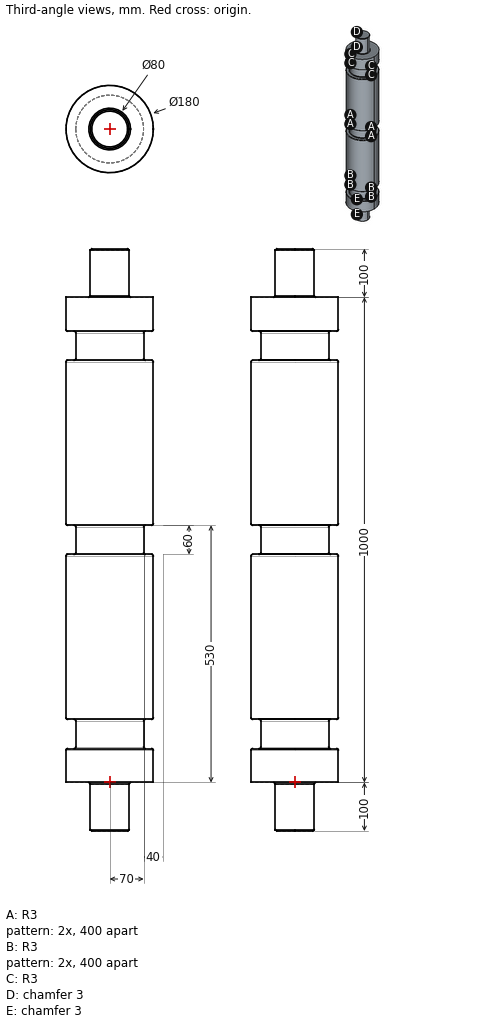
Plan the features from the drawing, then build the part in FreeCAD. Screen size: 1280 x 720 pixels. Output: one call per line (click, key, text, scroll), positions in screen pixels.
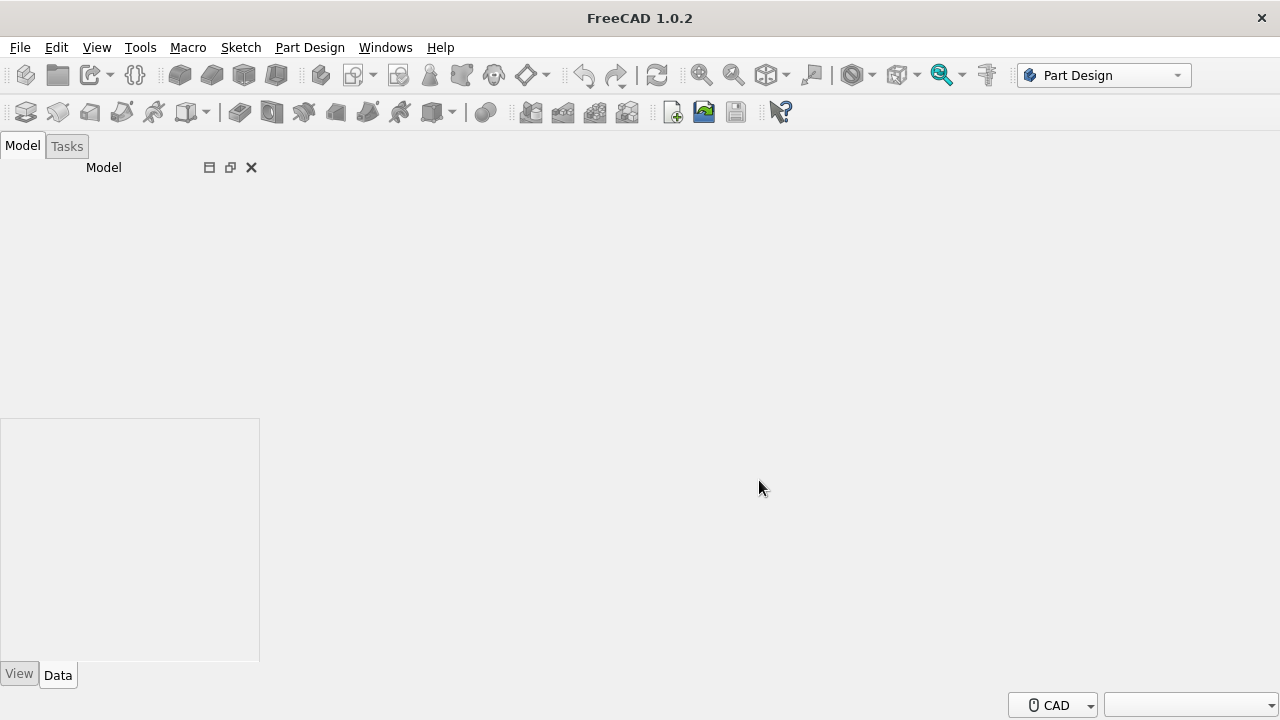
click(672, 112)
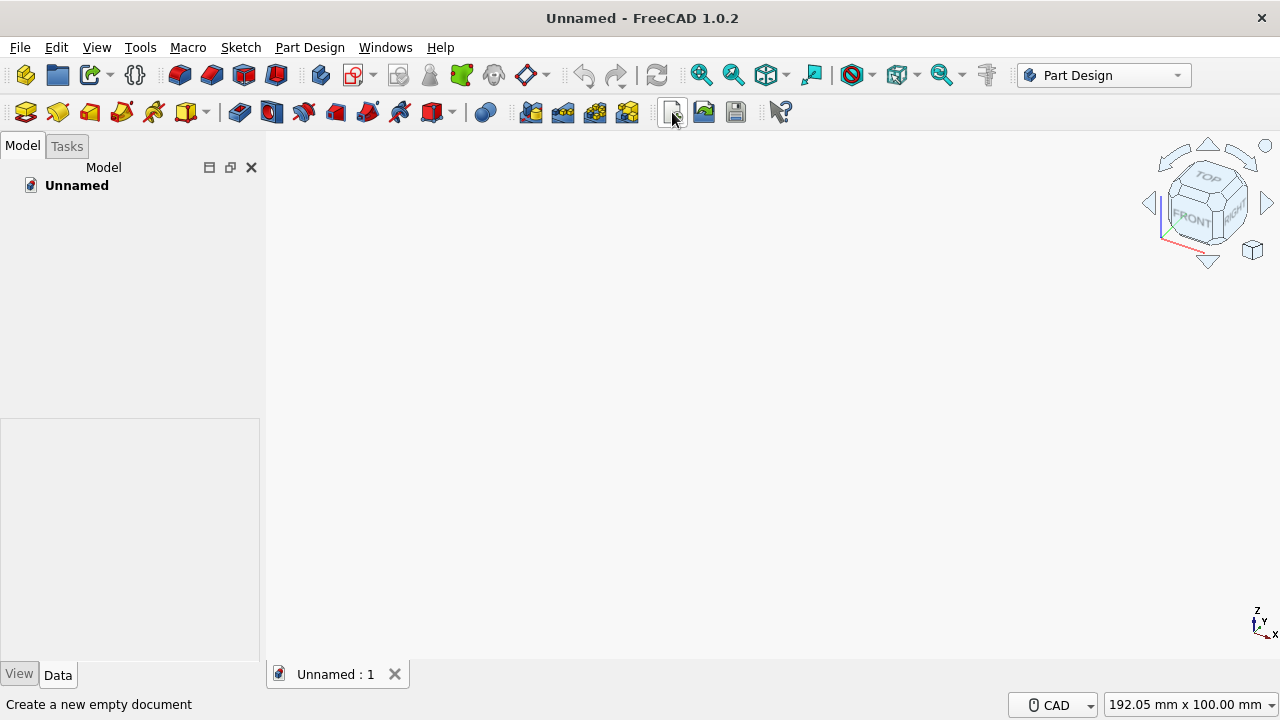
click(354, 76)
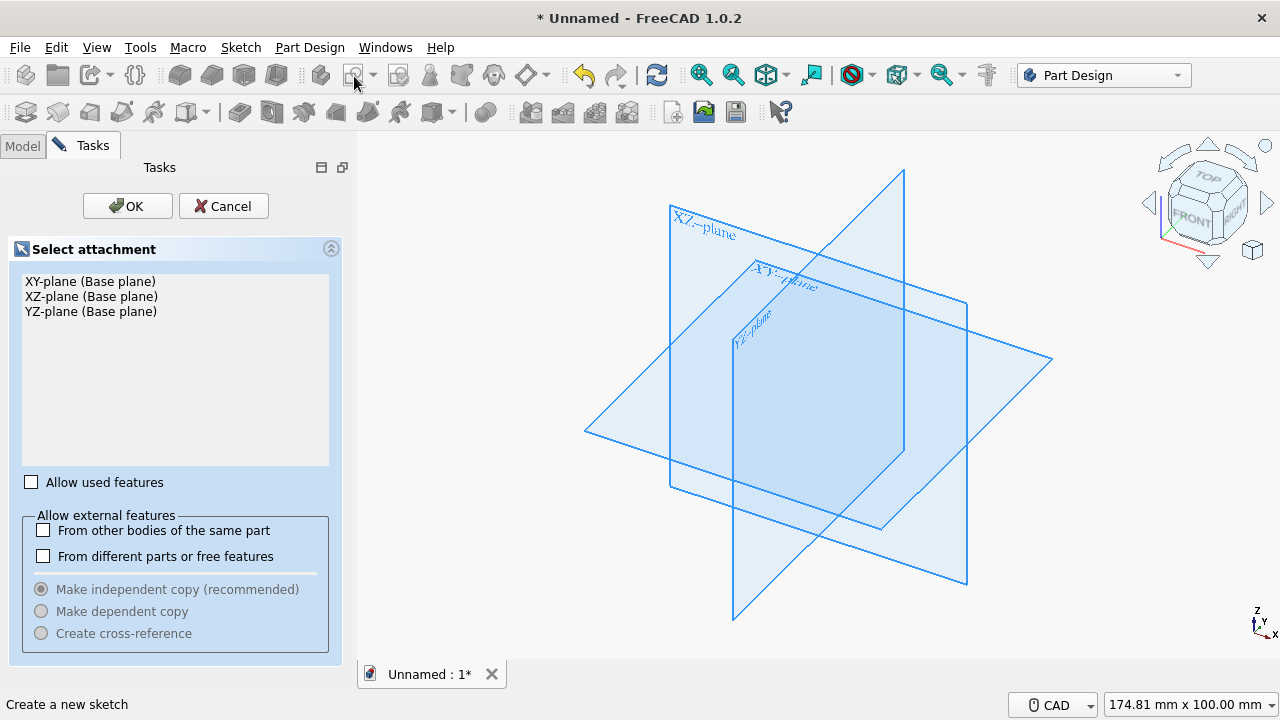
click(82, 282)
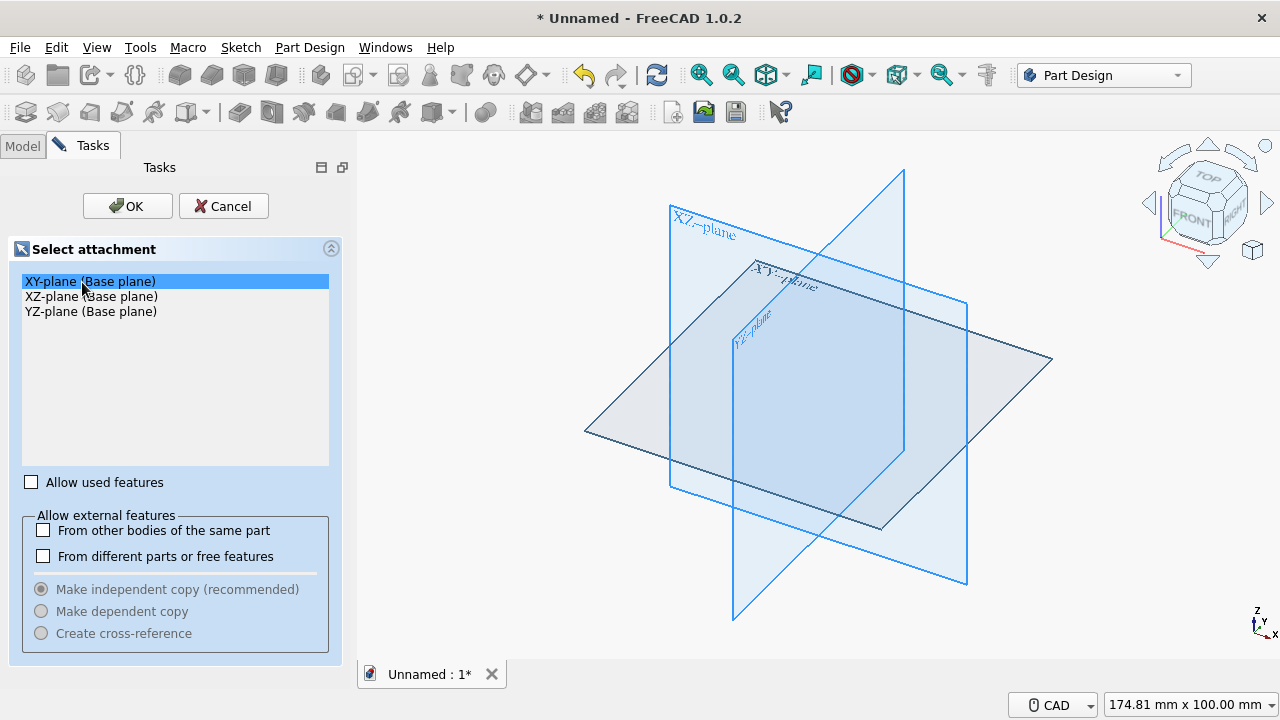
click(128, 206)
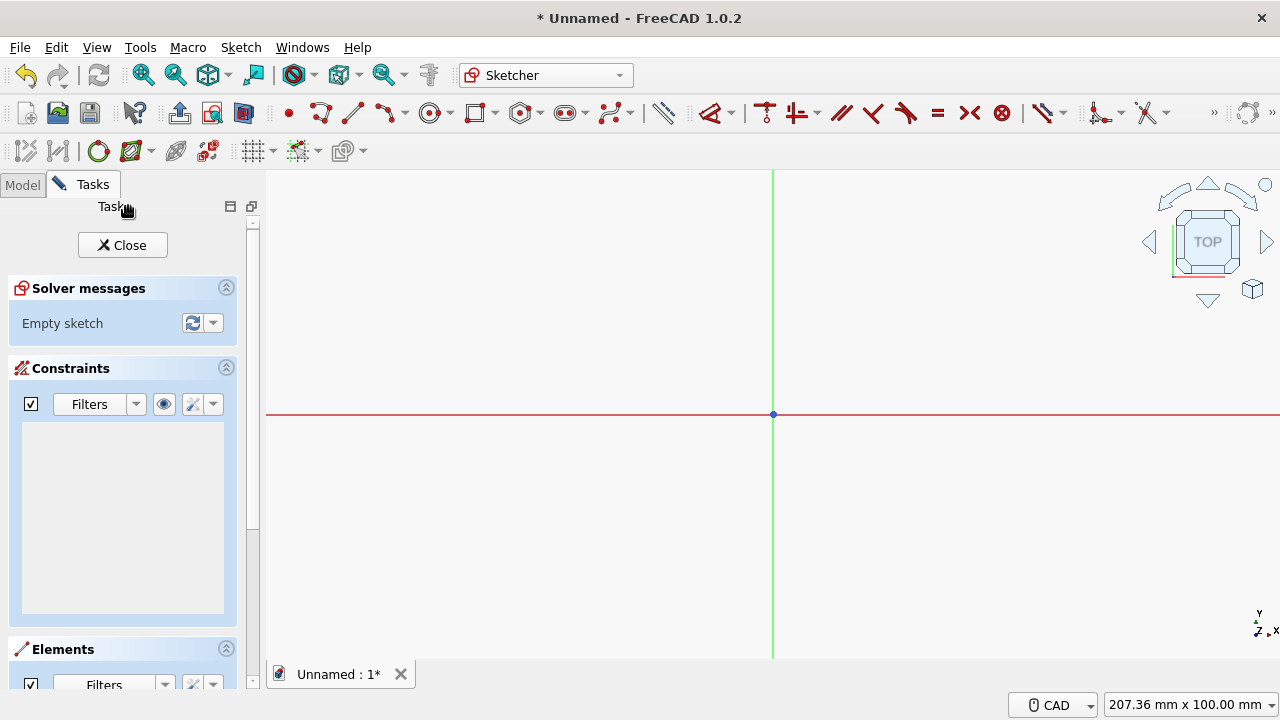
scroll(665, 414, down, 5)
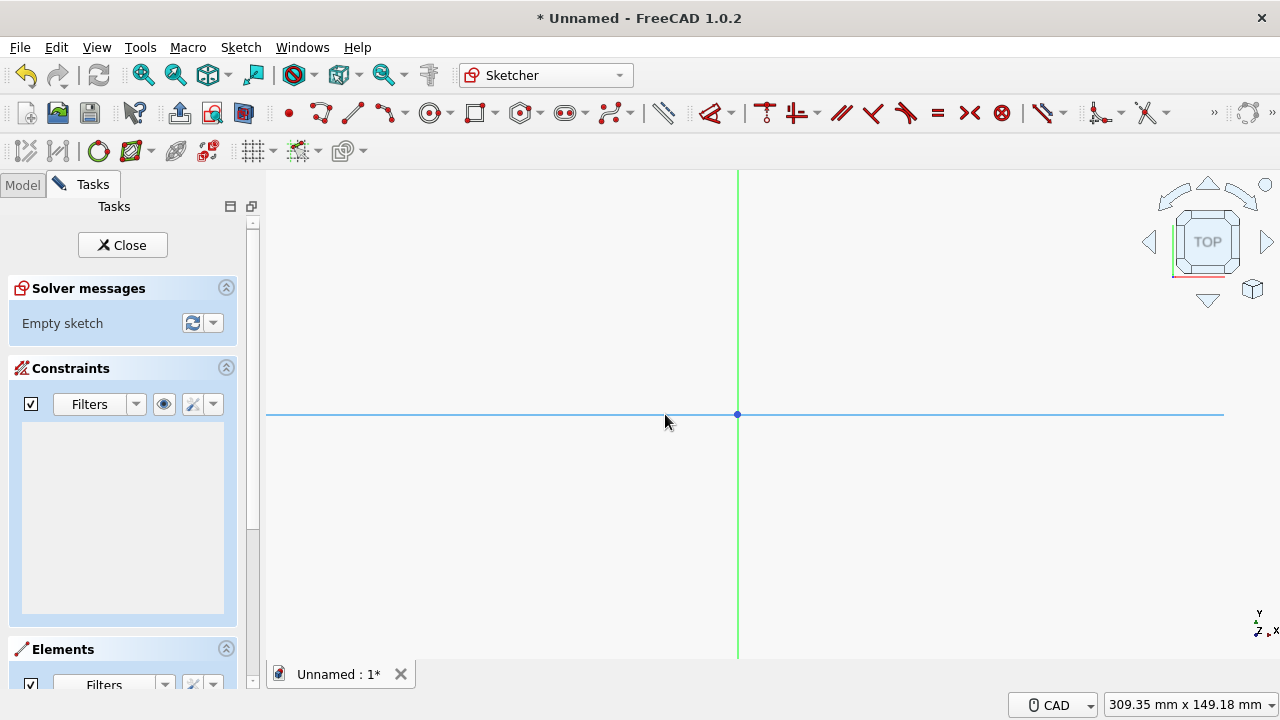
click(430, 114)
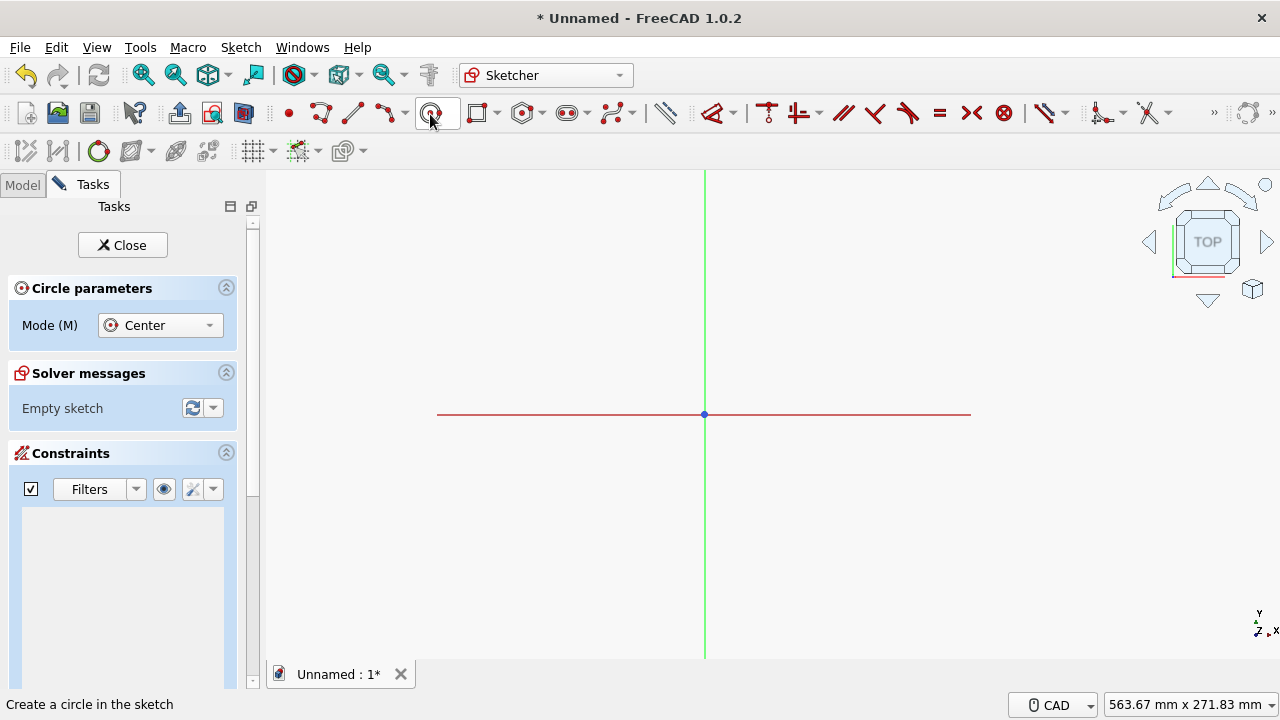
click(705, 414)
move(819, 300)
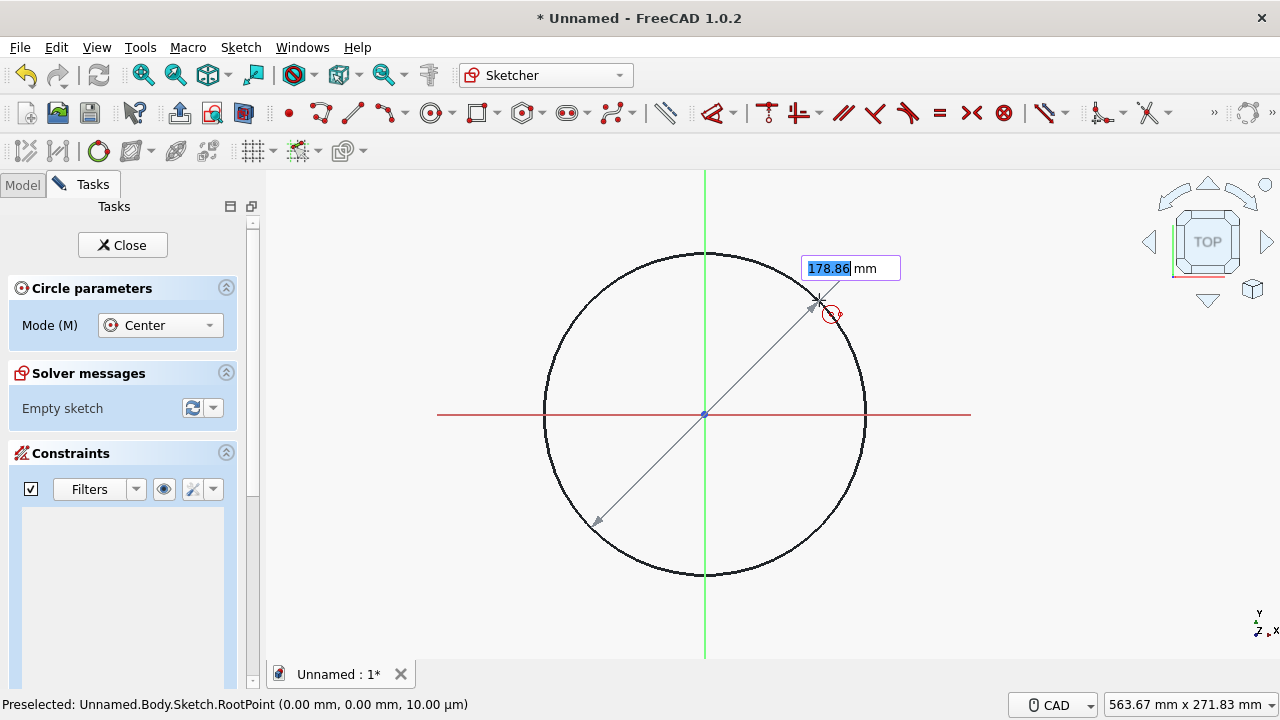
text(180)
key(Return)
key(Escape)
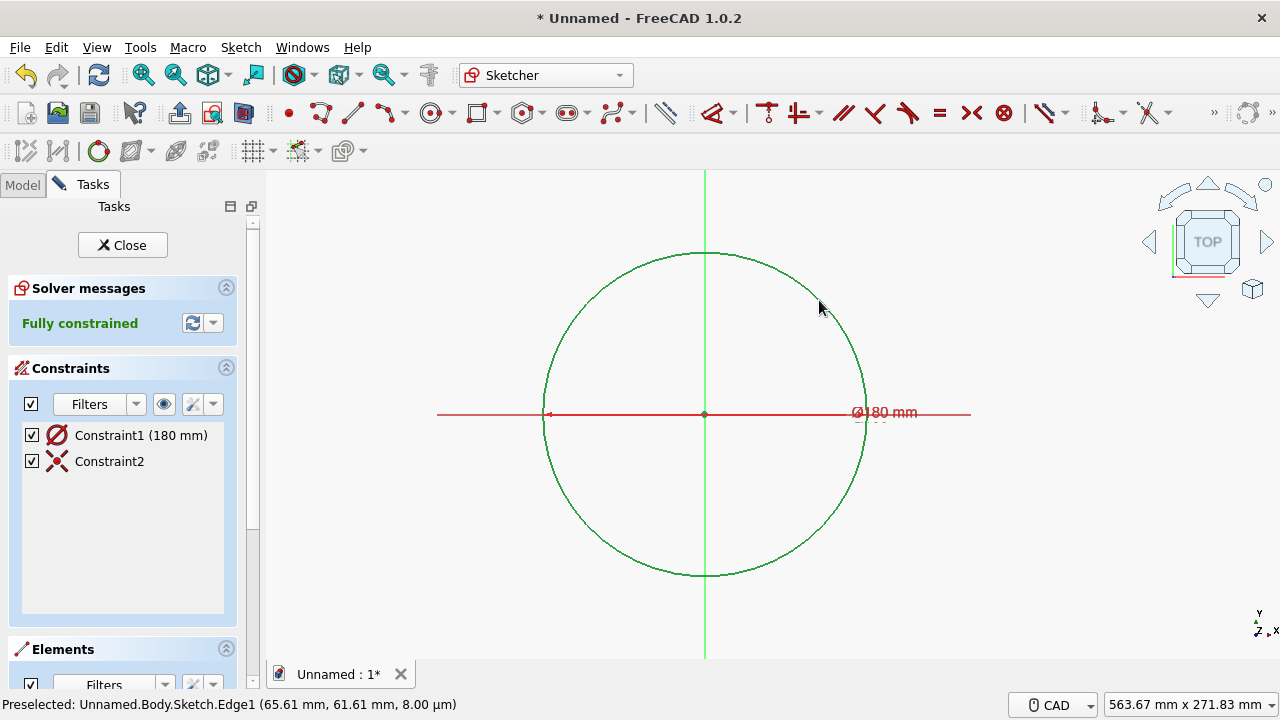
click(123, 245)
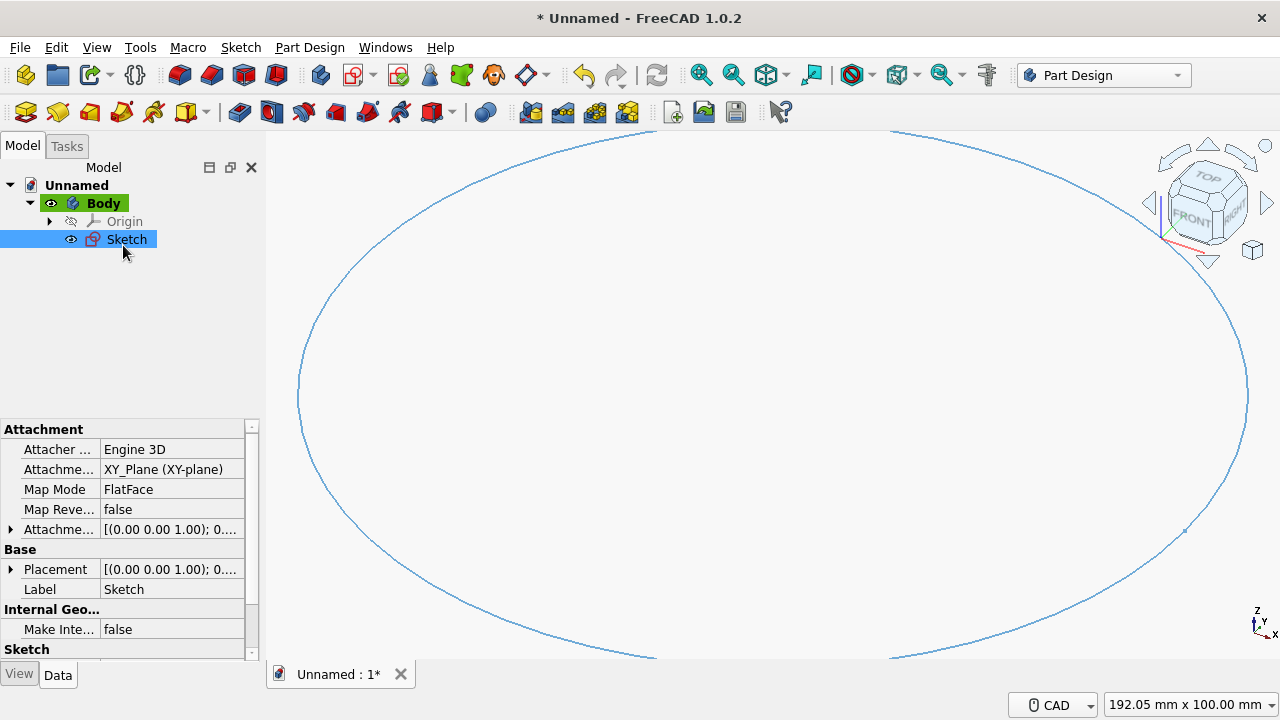
click(26, 112)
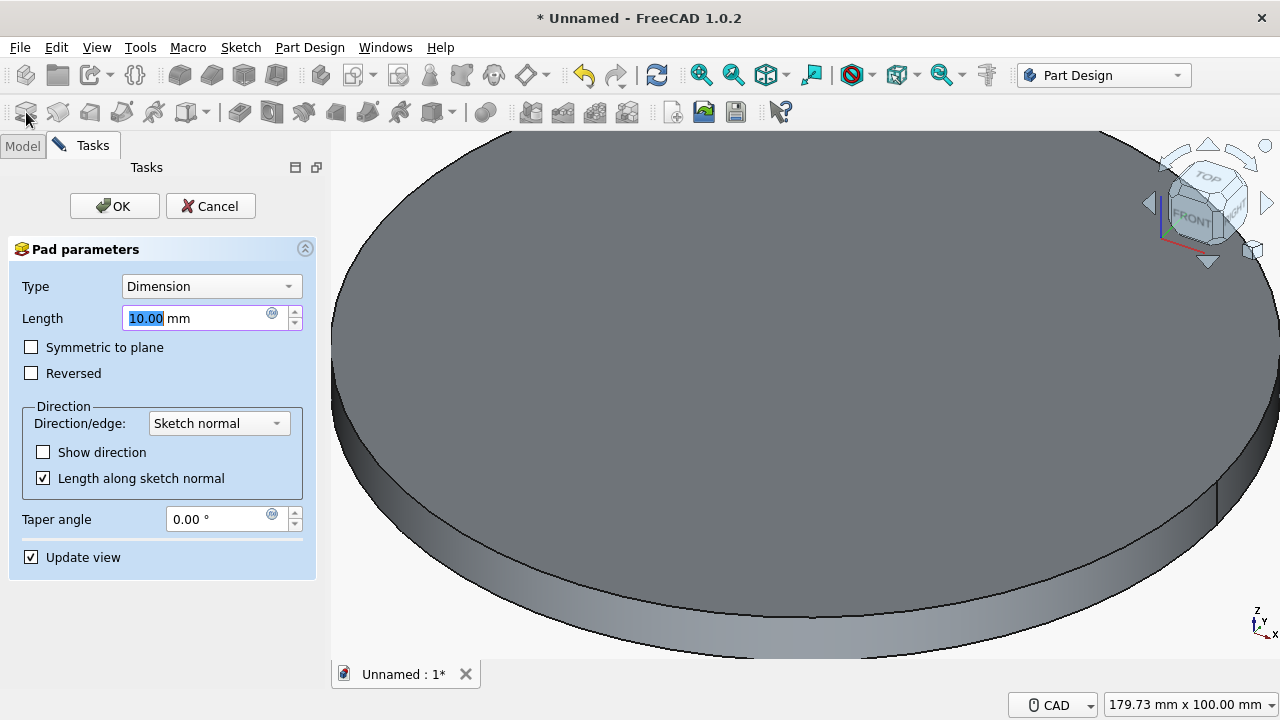
text(1000)
key(Tab)